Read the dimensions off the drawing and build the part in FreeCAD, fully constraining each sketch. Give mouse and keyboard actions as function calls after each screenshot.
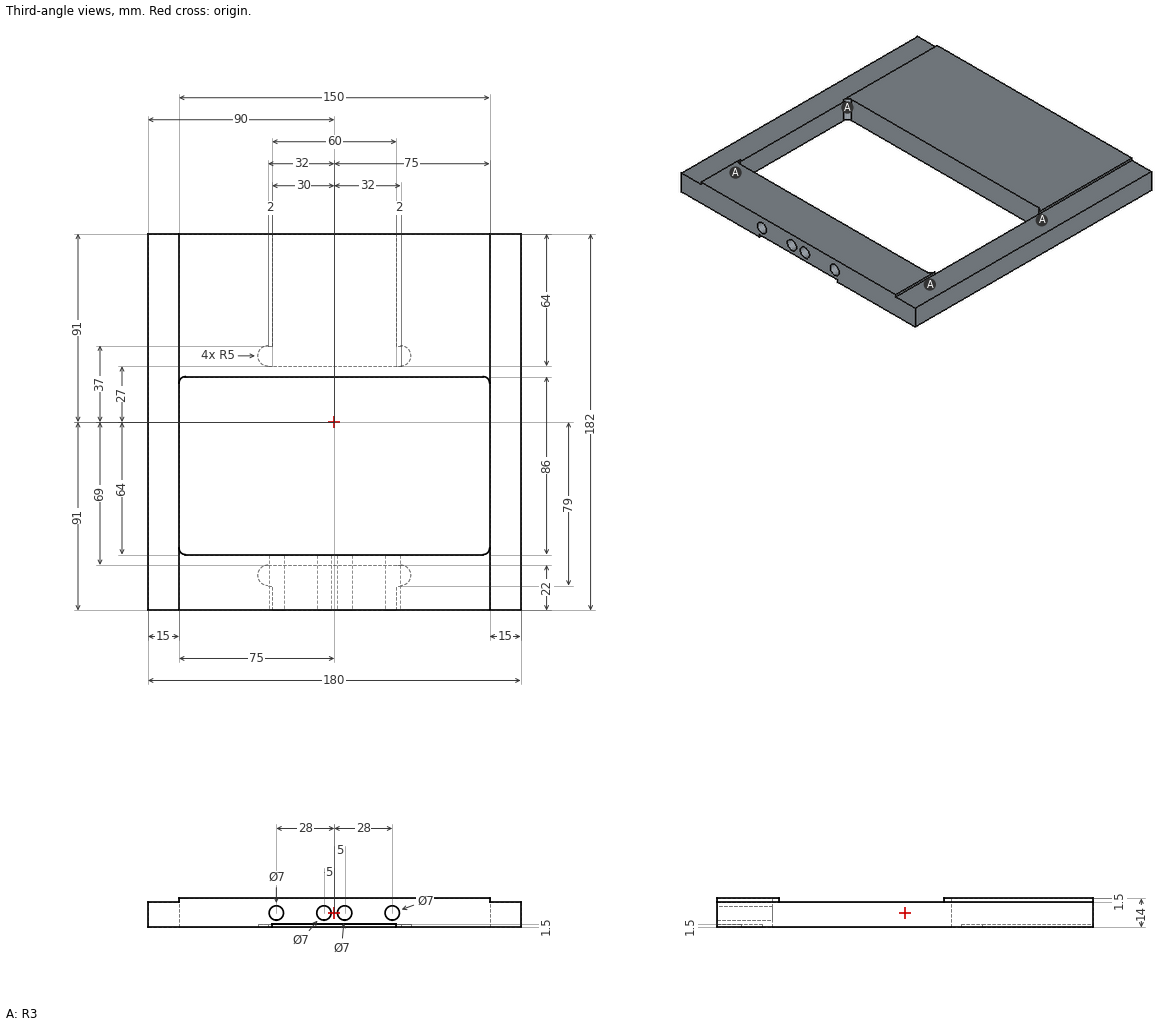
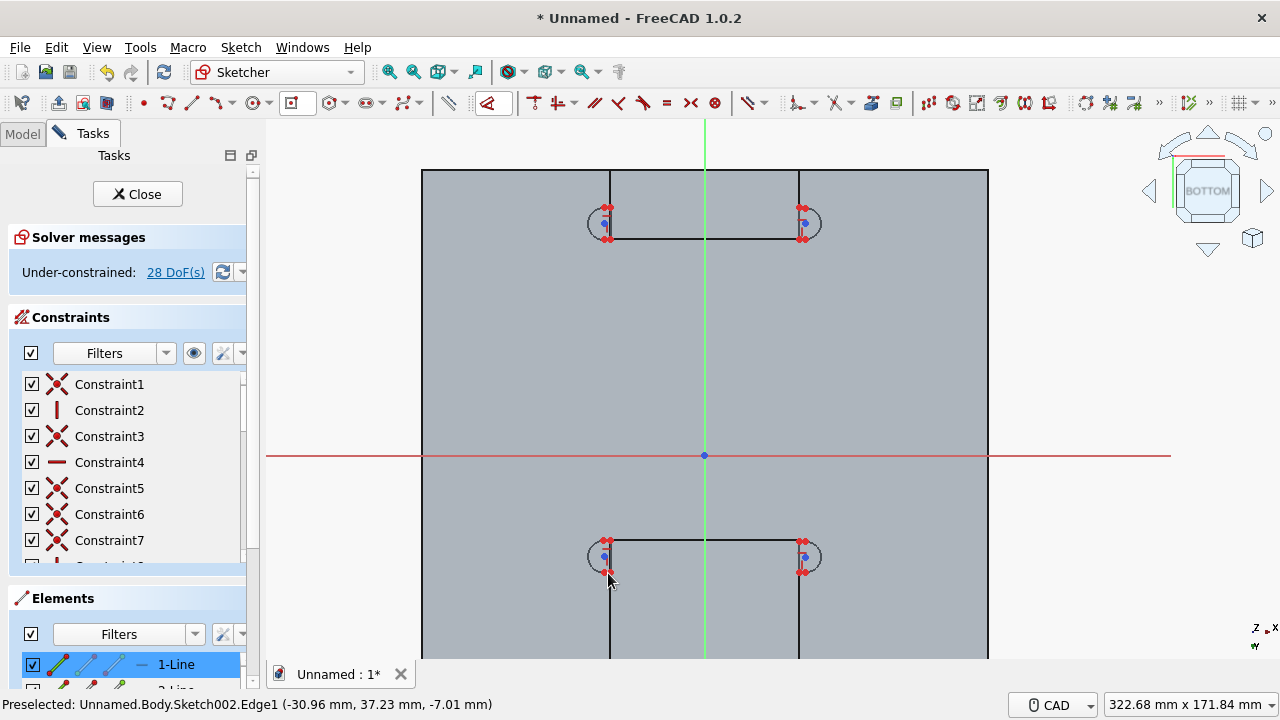
click(591, 547)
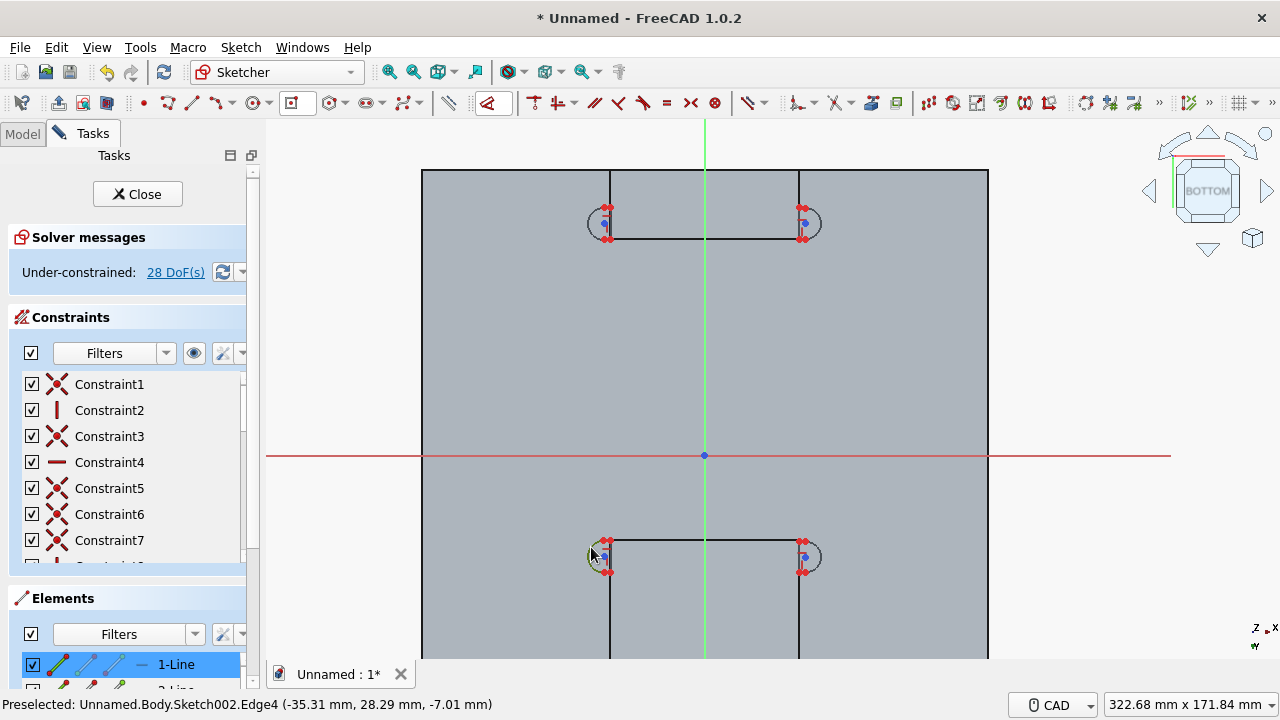
key(t)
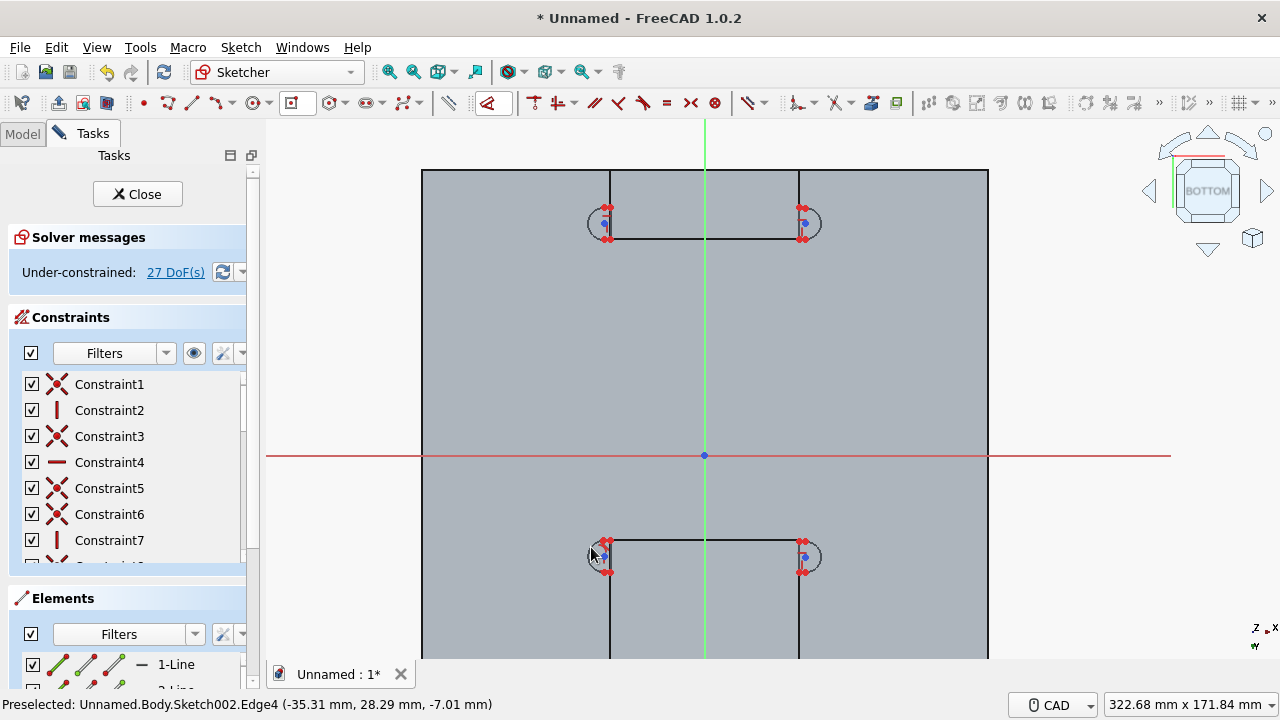
scroll(607, 541, up, 8)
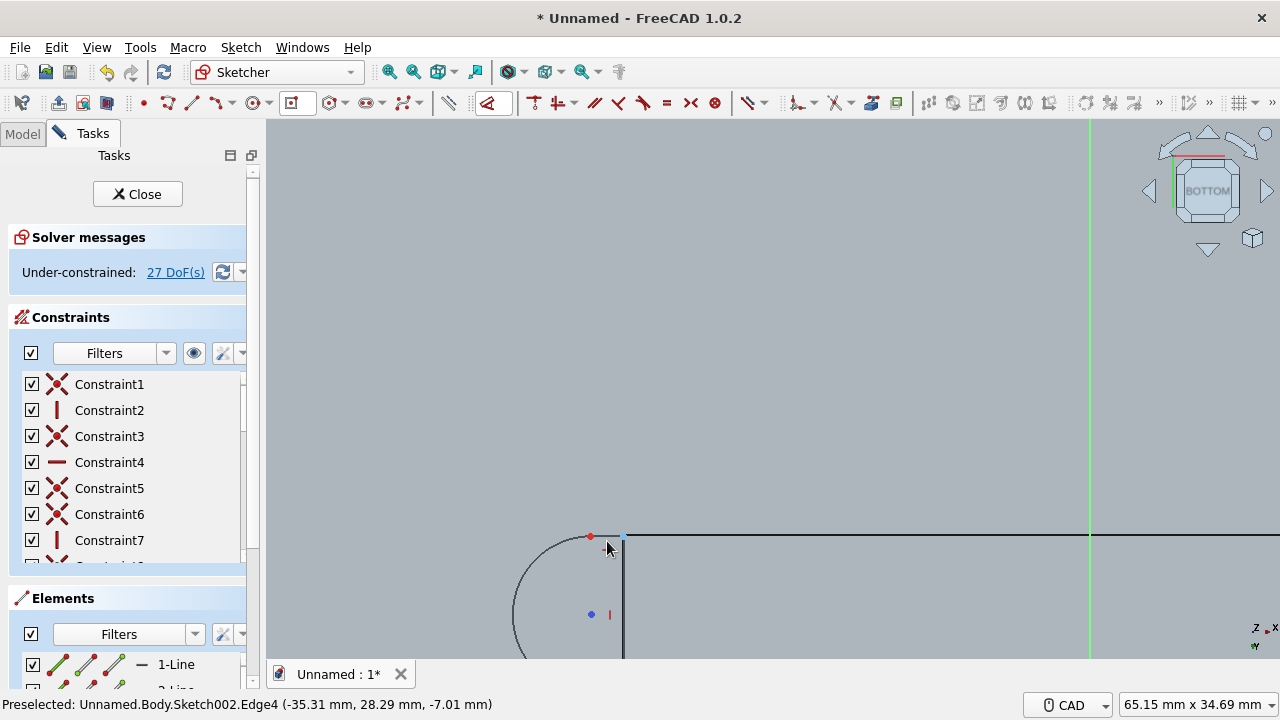
click(607, 536)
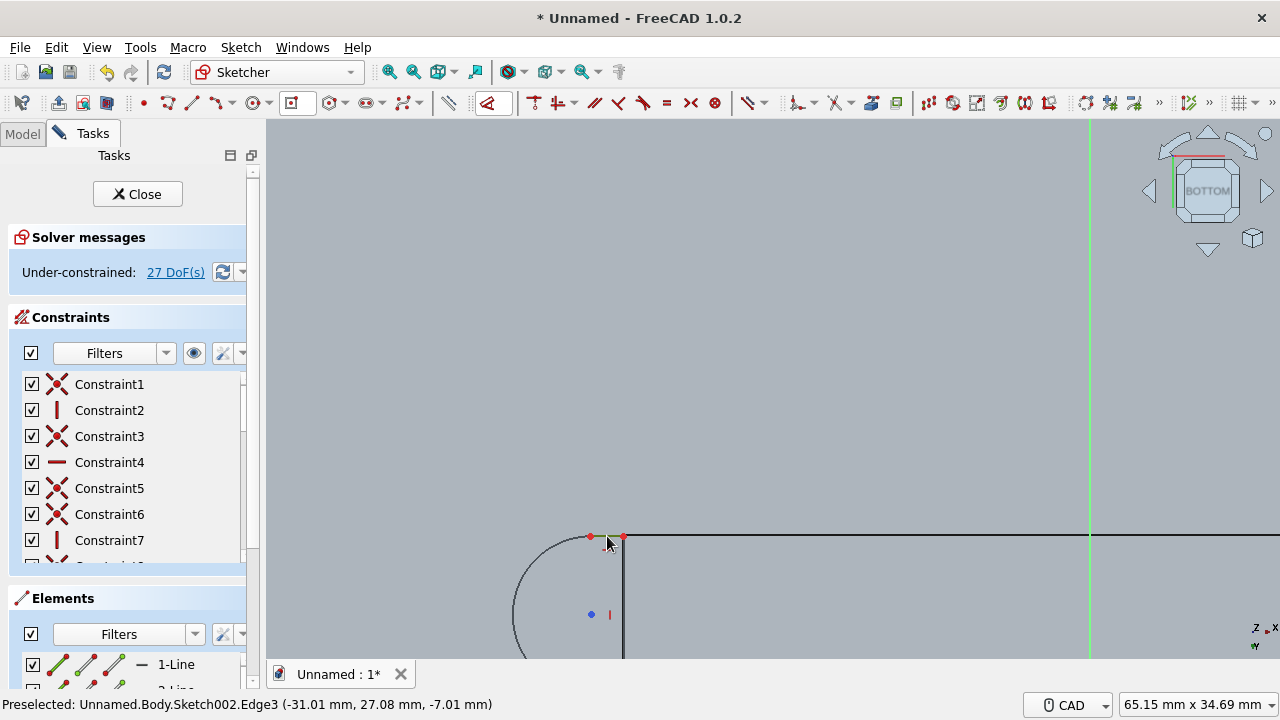
scroll(607, 541, down, 8)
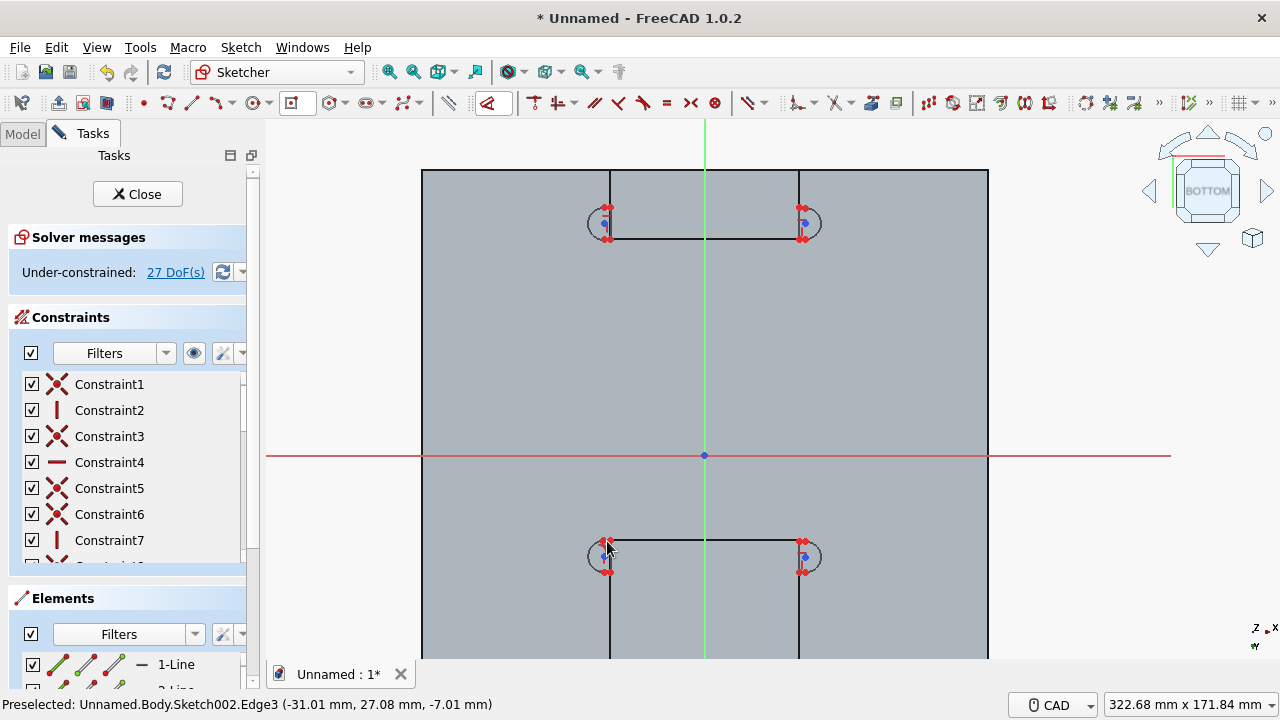
click(591, 547)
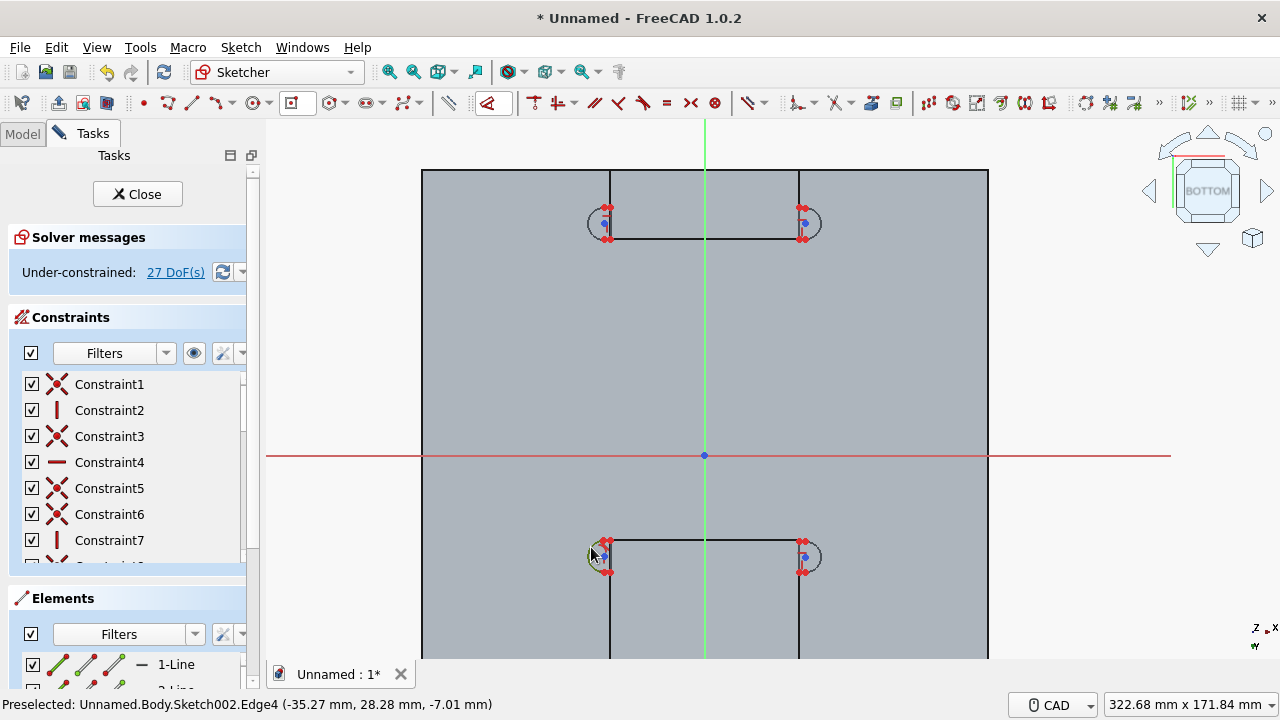
key(t)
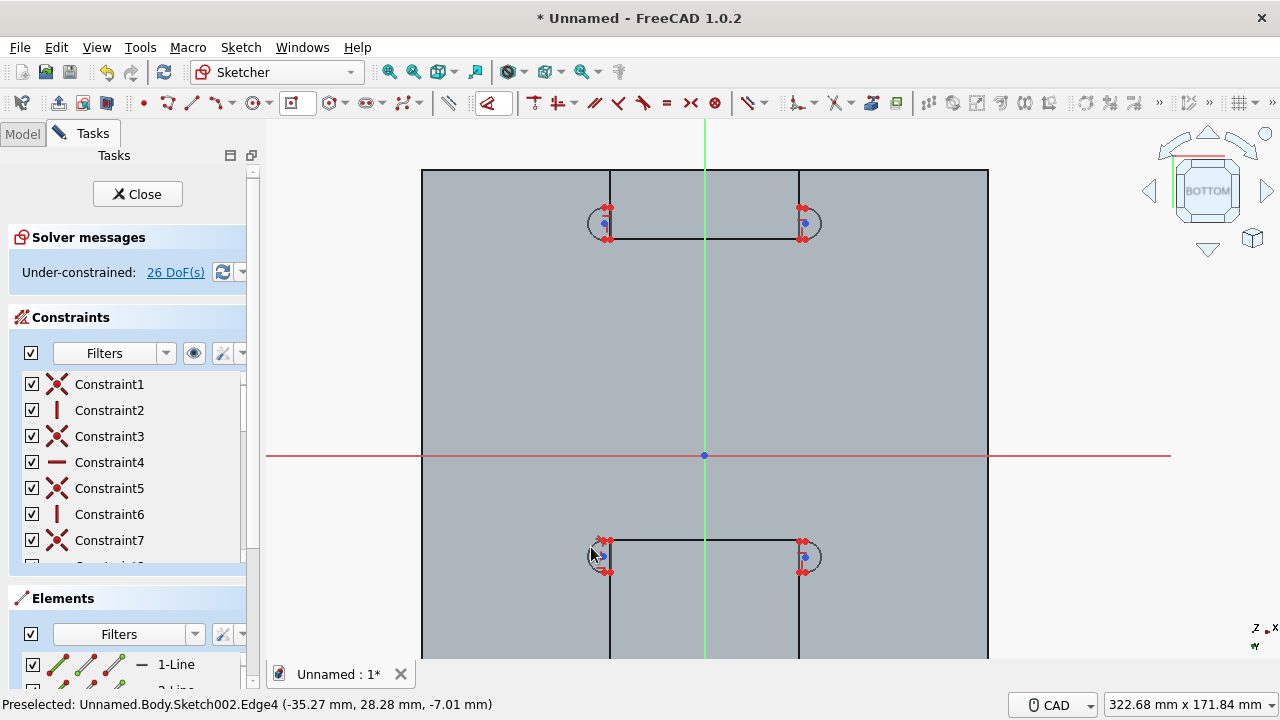
scroll(802, 542, up, 8)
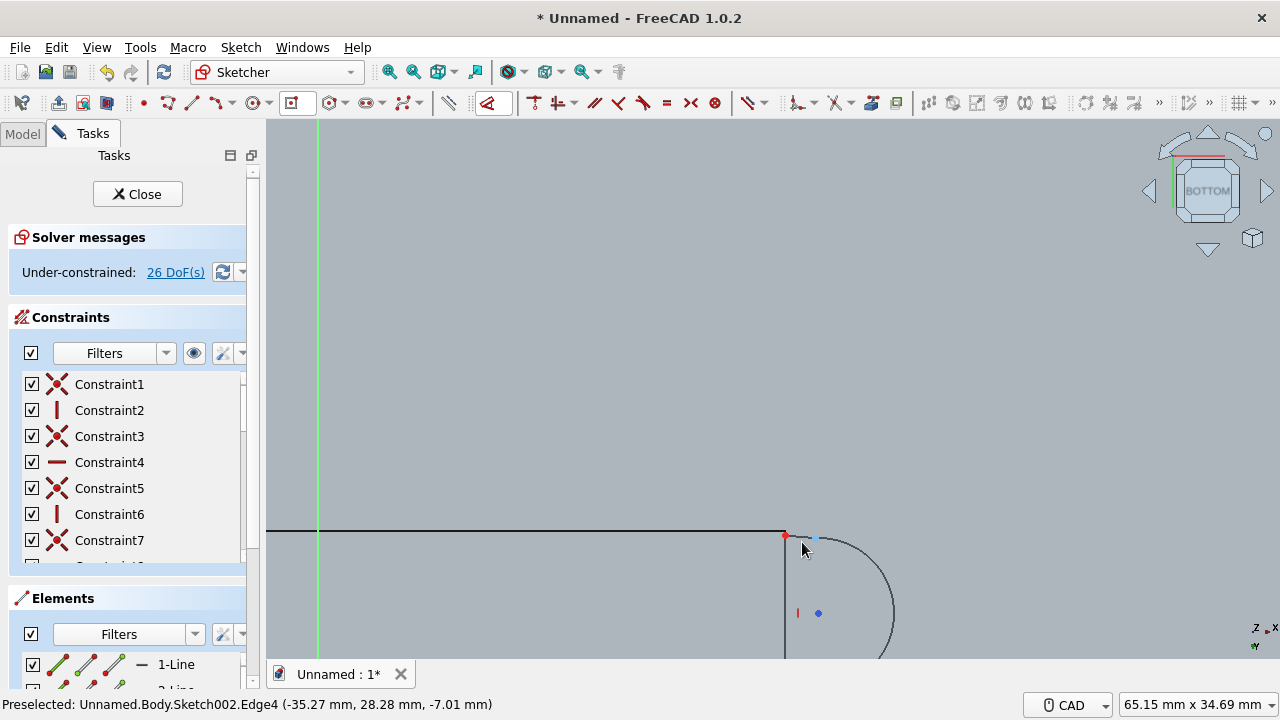
click(800, 537)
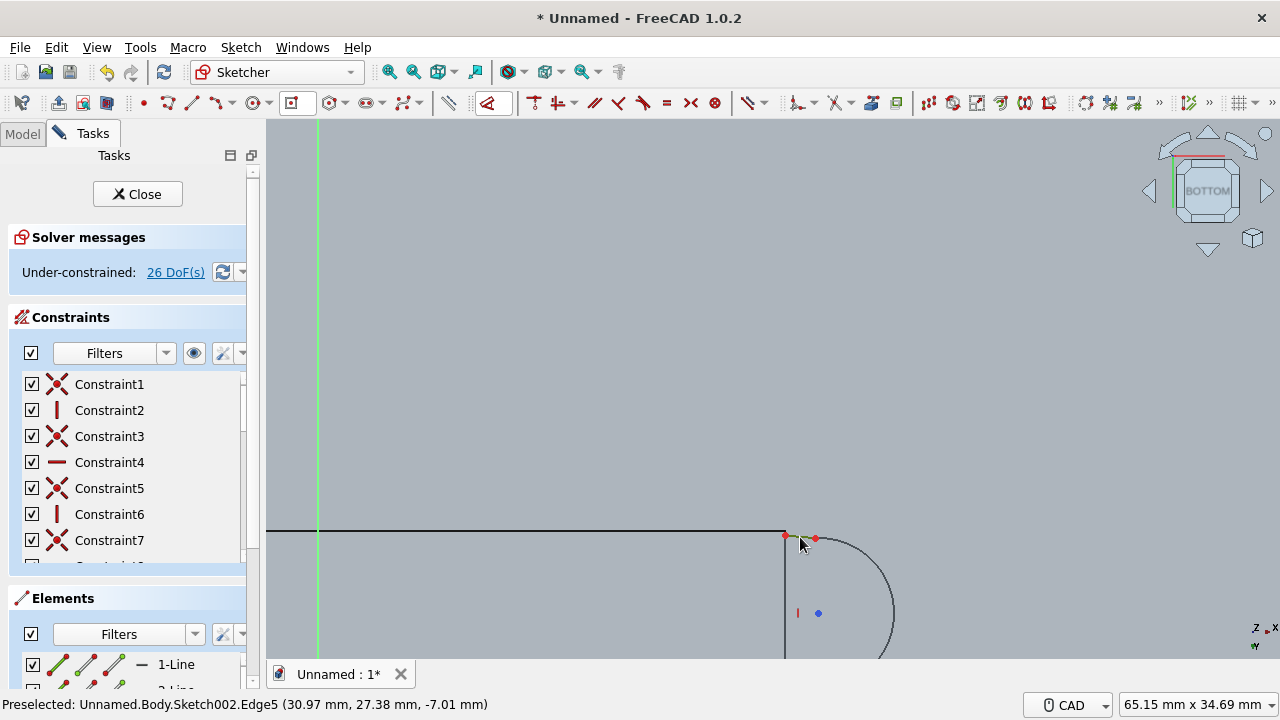
scroll(802, 542, down, 8)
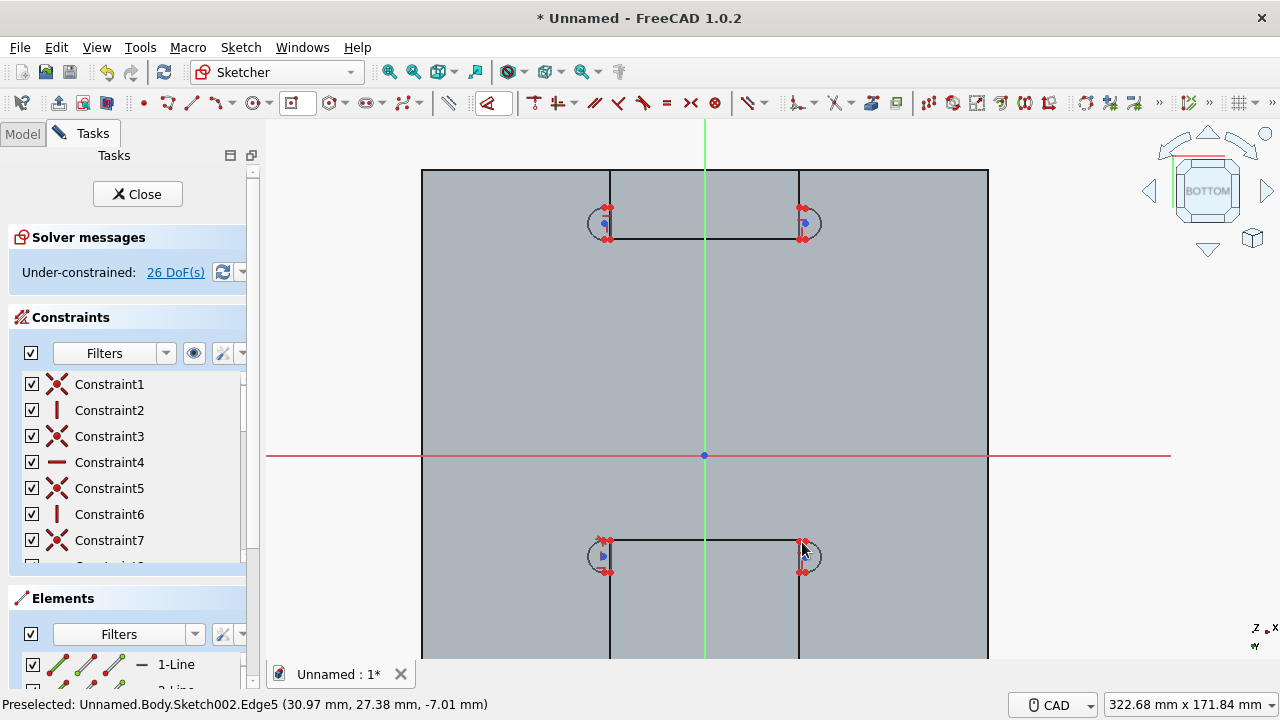
click(818, 548)